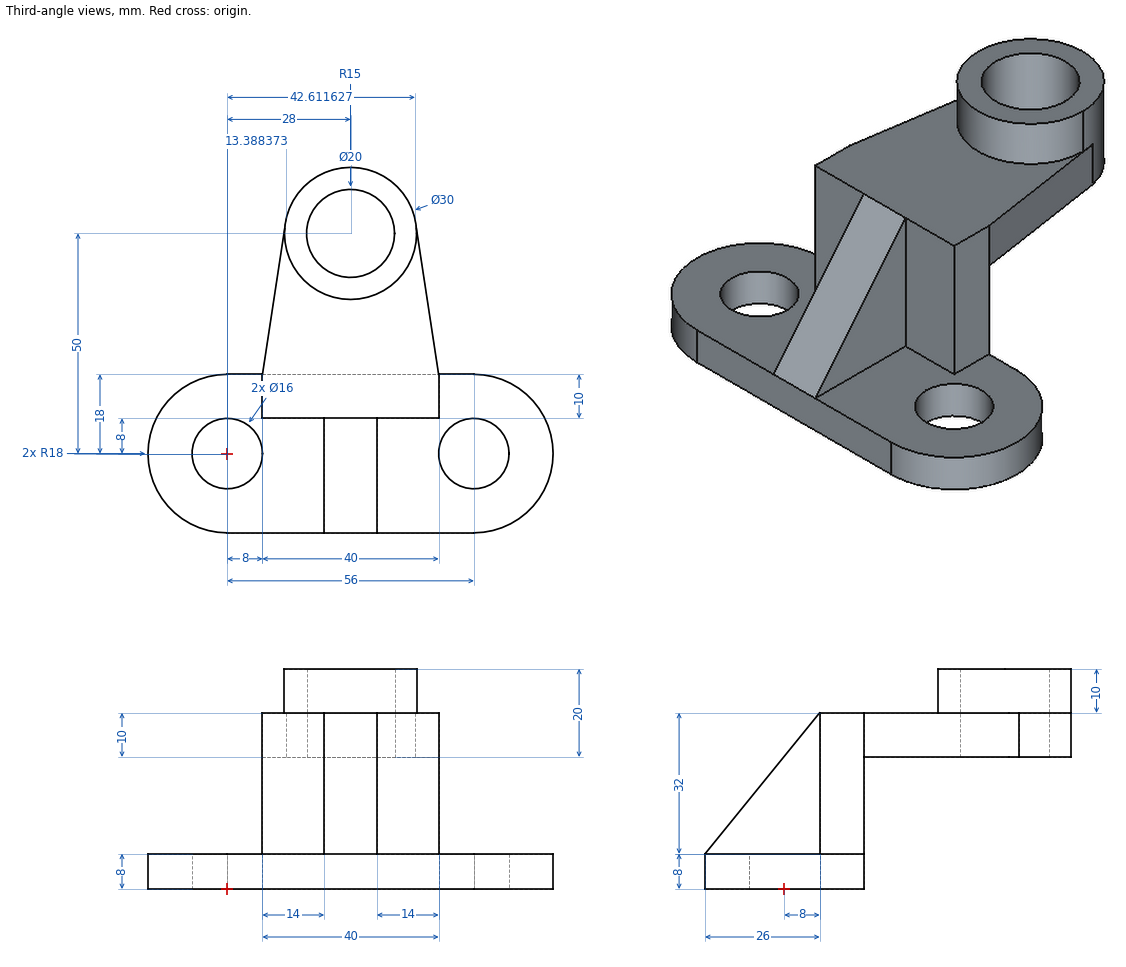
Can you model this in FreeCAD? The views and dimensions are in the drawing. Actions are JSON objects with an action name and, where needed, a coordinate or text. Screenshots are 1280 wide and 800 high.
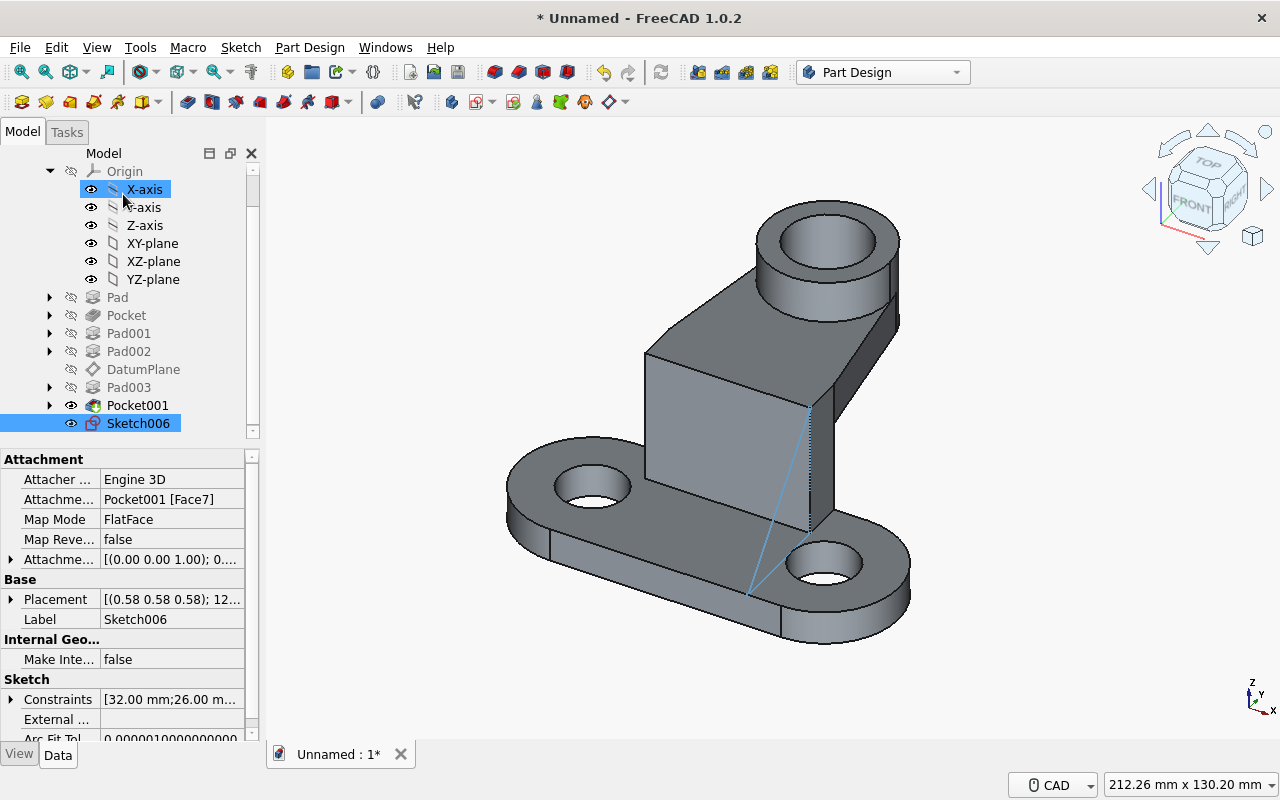
{"action": "left_click", "coordinate": [22, 102]}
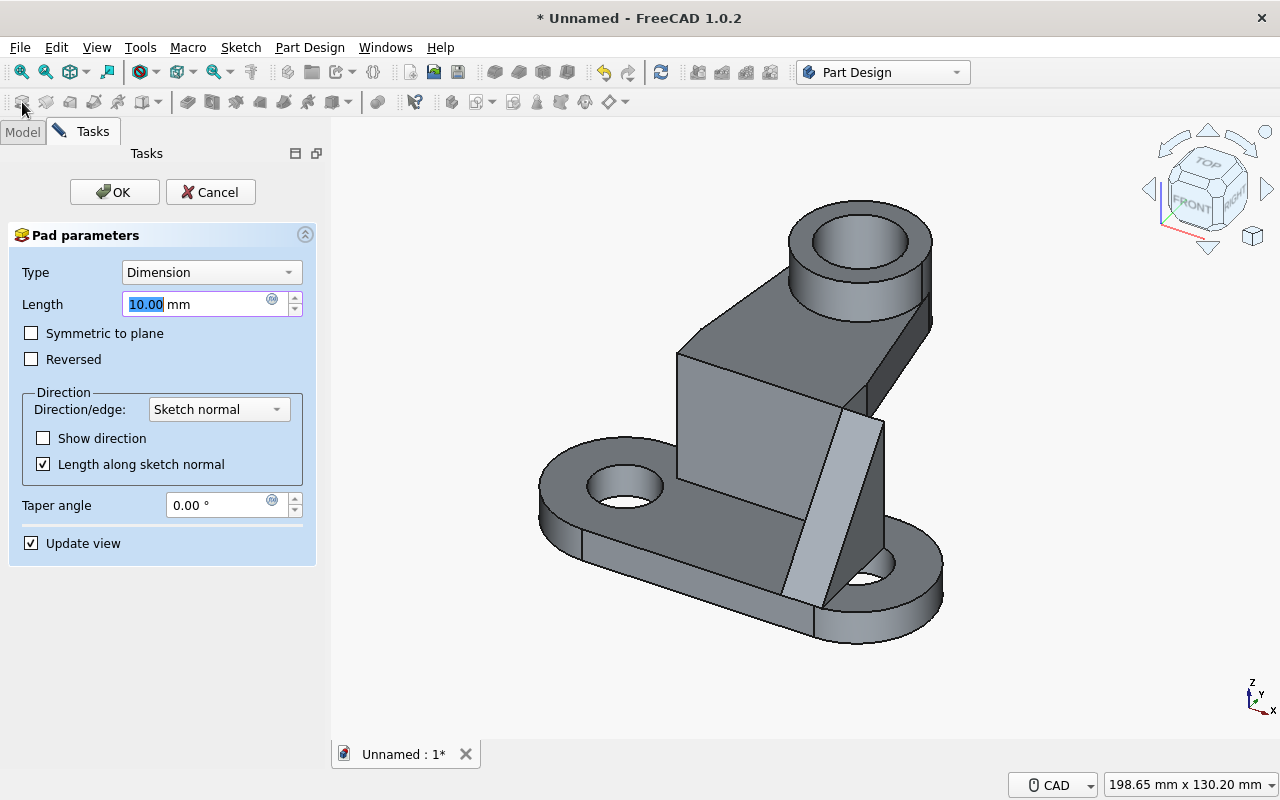
{"action": "type", "text": "40"}
{"action": "key", "text": "Tab"}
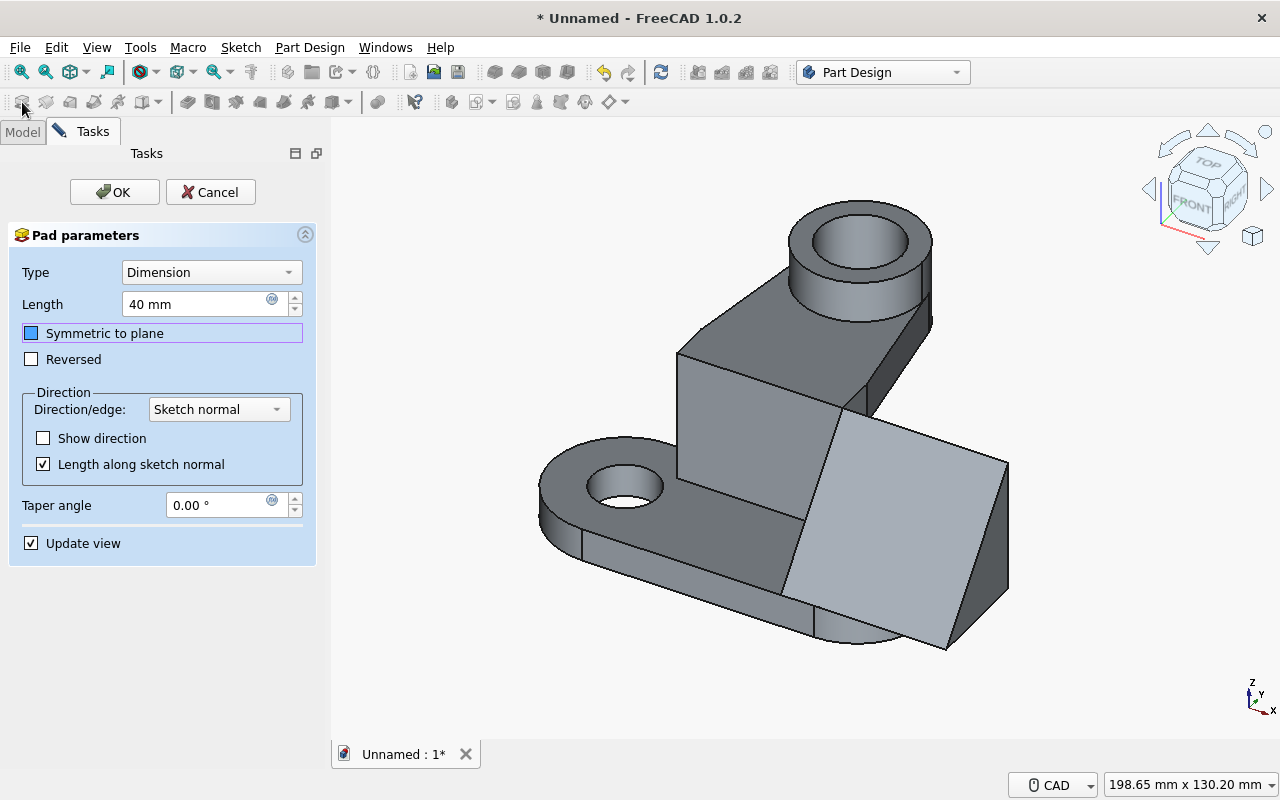
{"action": "left_click", "coordinate": [30, 359]}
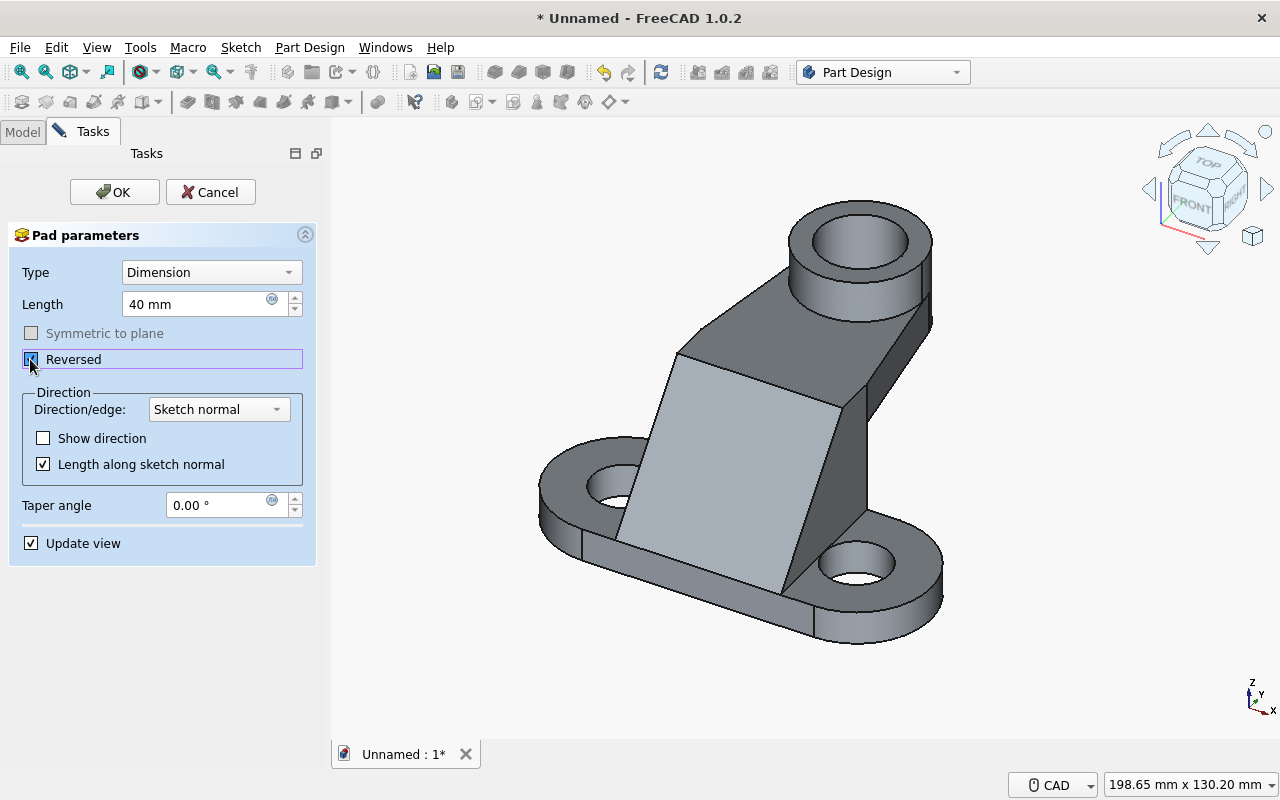
{"action": "left_click", "coordinate": [115, 192]}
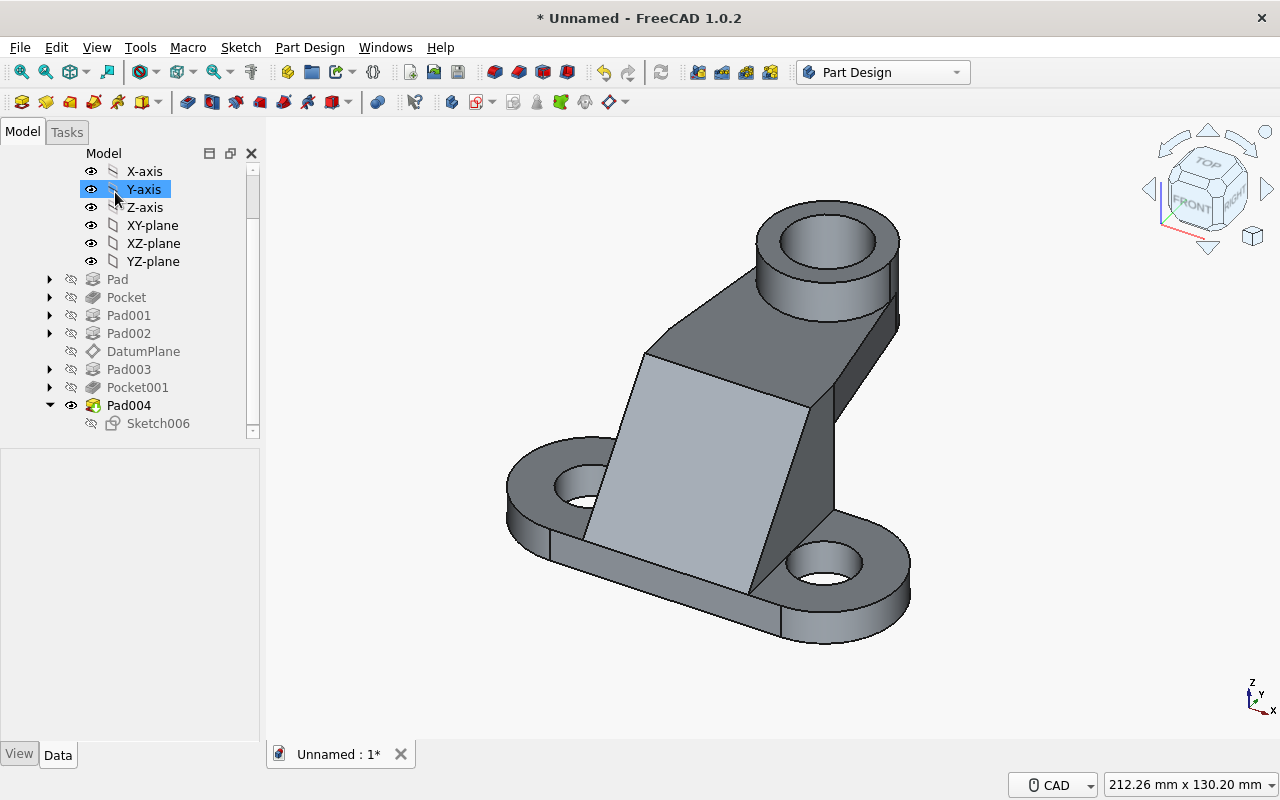
{"action": "left_click", "coordinate": [804, 494]}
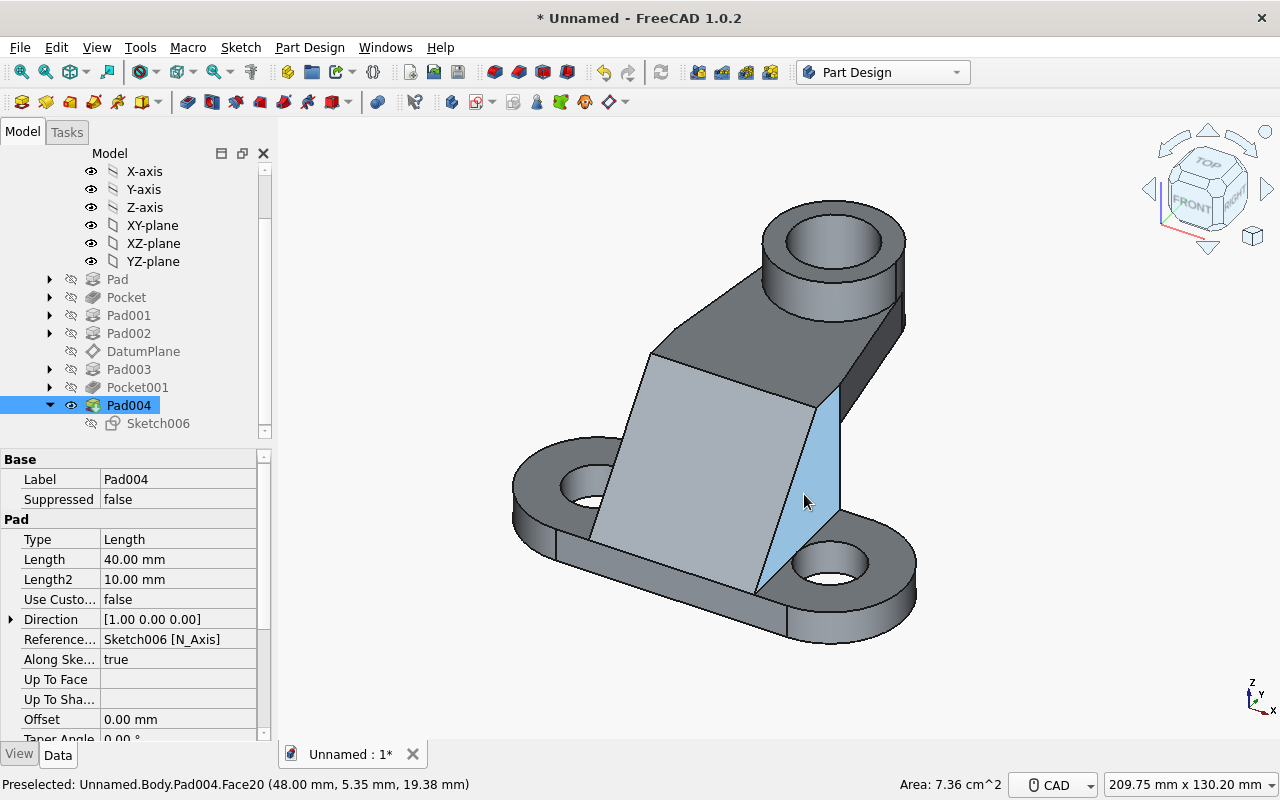
{"action": "left_click", "coordinate": [476, 102]}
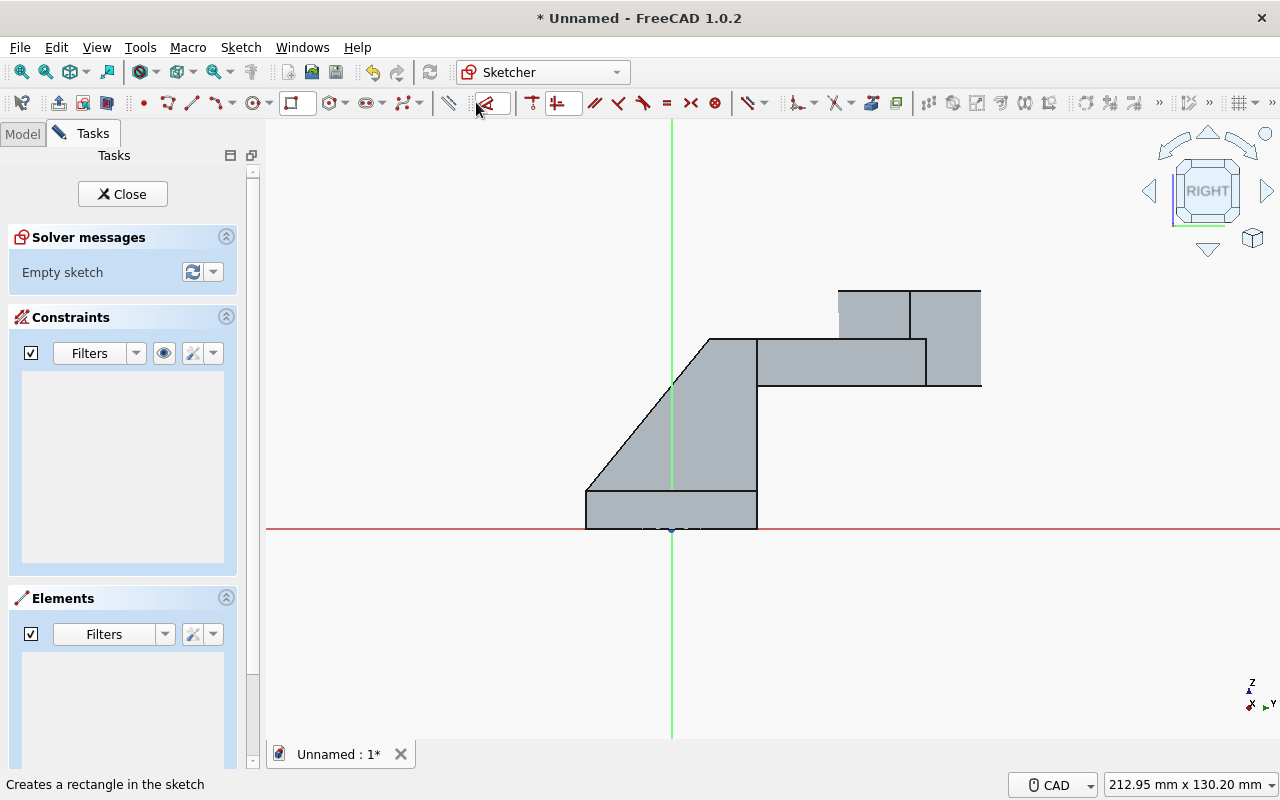
{"action": "scroll", "coordinate": [602, 438], "scroll_direction": "up", "scroll_amount": 4}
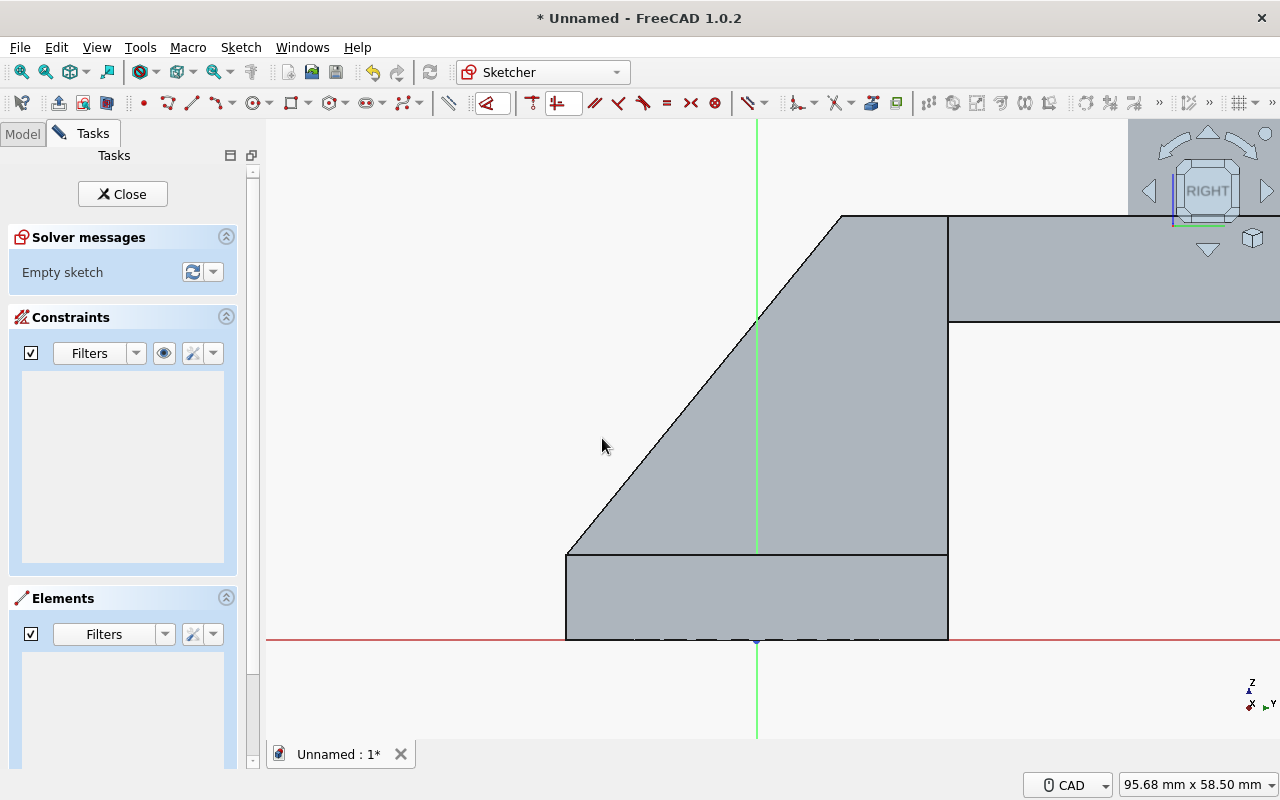
{"action": "left_click", "coordinate": [168, 104]}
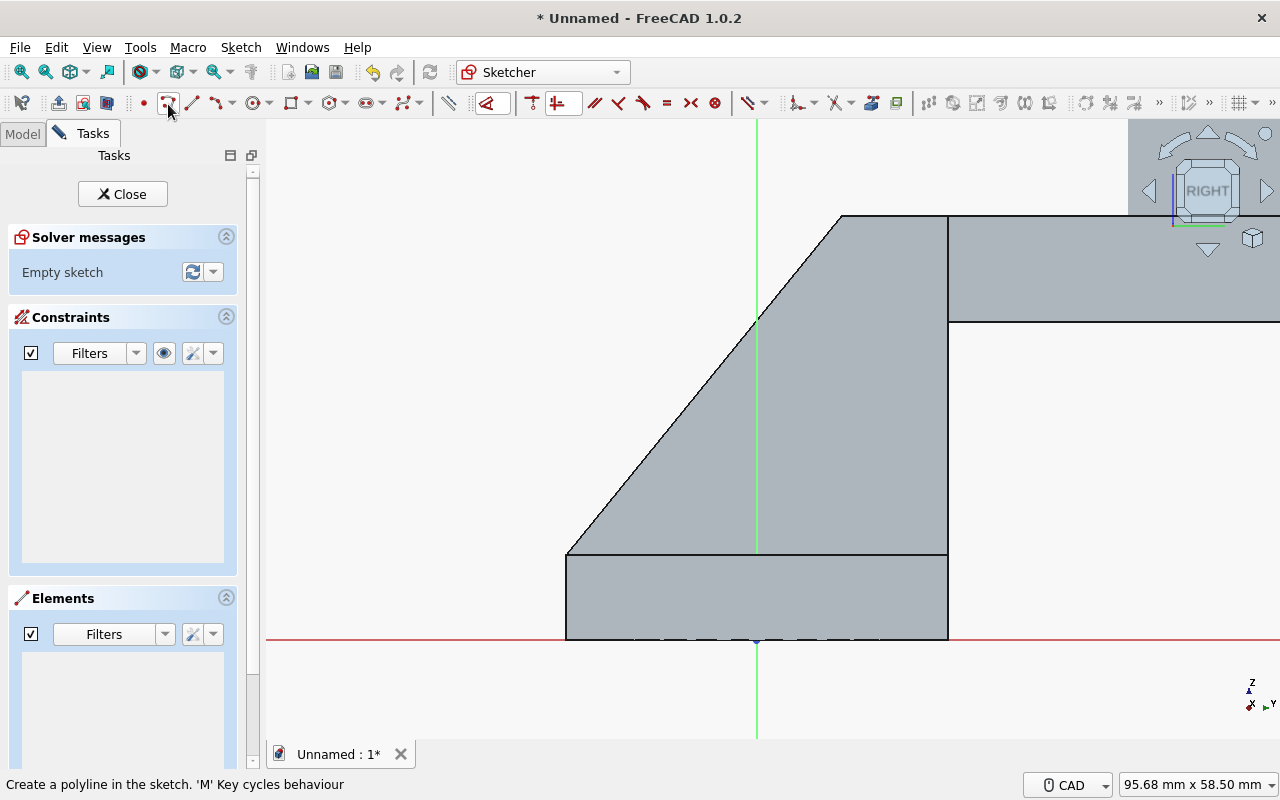
{"action": "left_click", "coordinate": [842, 555]}
{"action": "left_click", "coordinate": [842, 216]}
{"action": "left_click", "coordinate": [566, 555]}
{"action": "left_click", "coordinate": [842, 556]}
{"action": "key", "text": "Escape"}
{"action": "key", "text": "Escape"}